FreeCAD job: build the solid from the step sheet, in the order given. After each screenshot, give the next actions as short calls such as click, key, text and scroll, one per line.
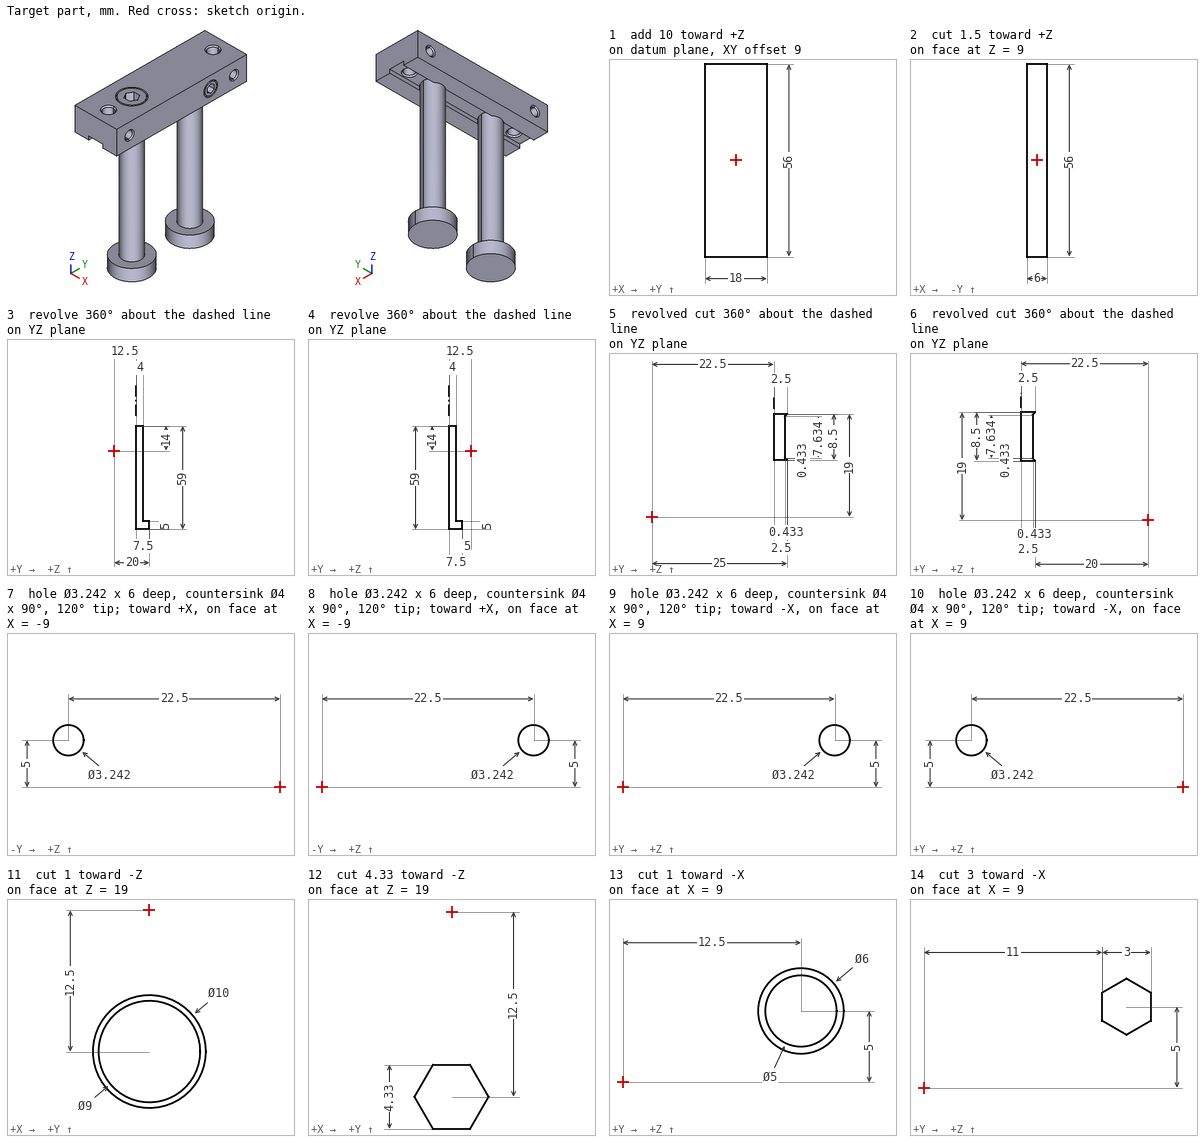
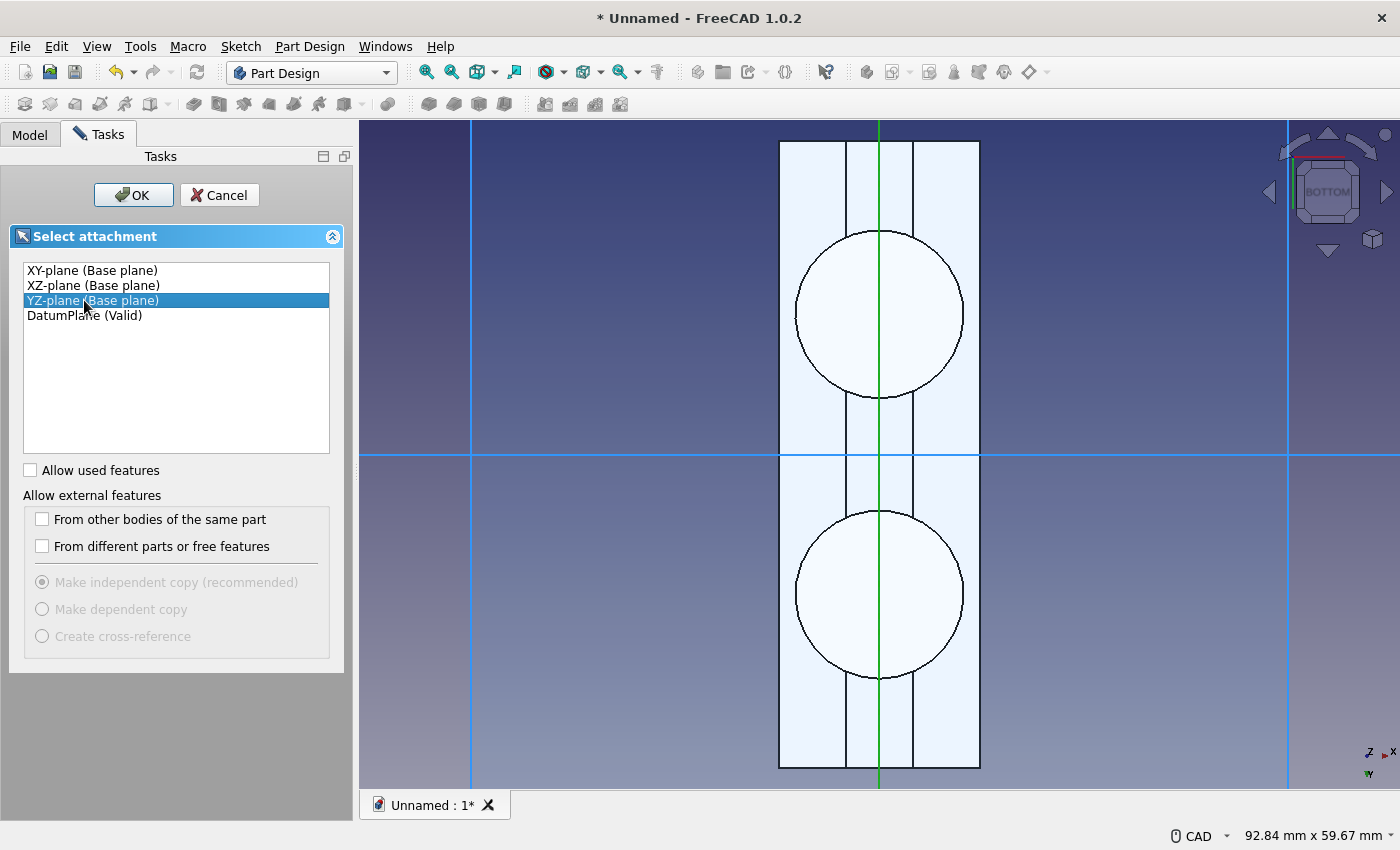
click(134, 195)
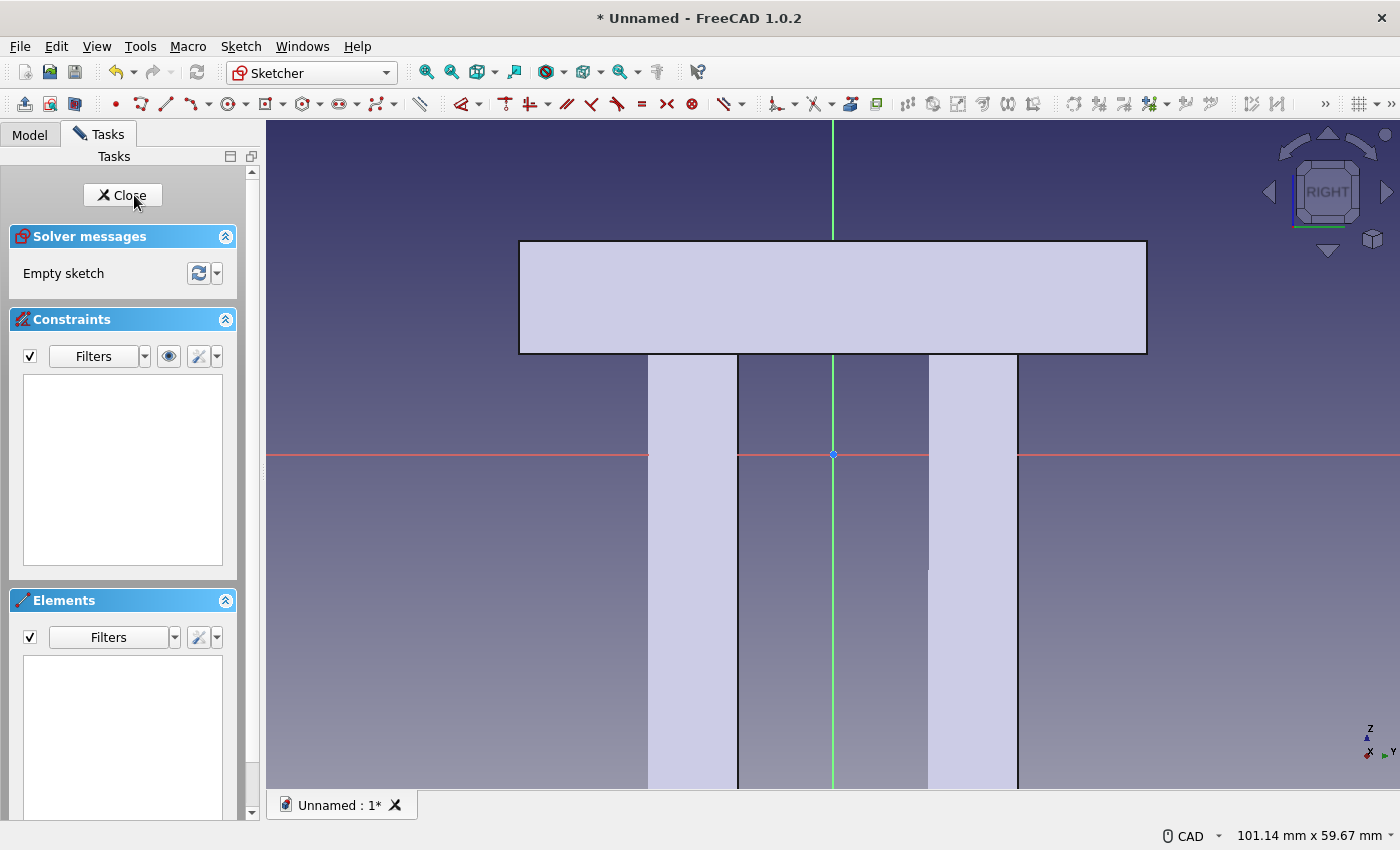
click(75, 104)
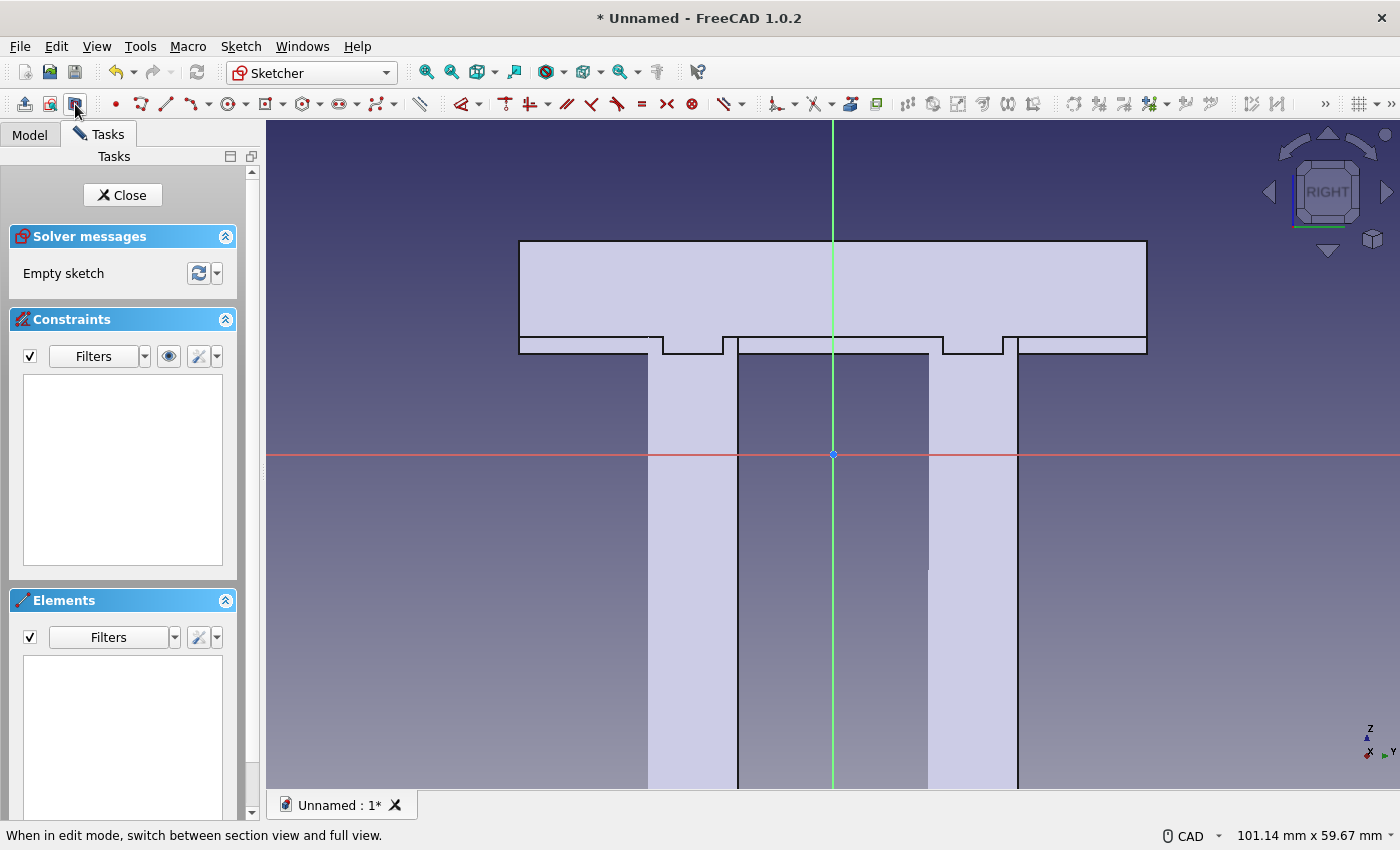
scroll(1227, 176, up, 3)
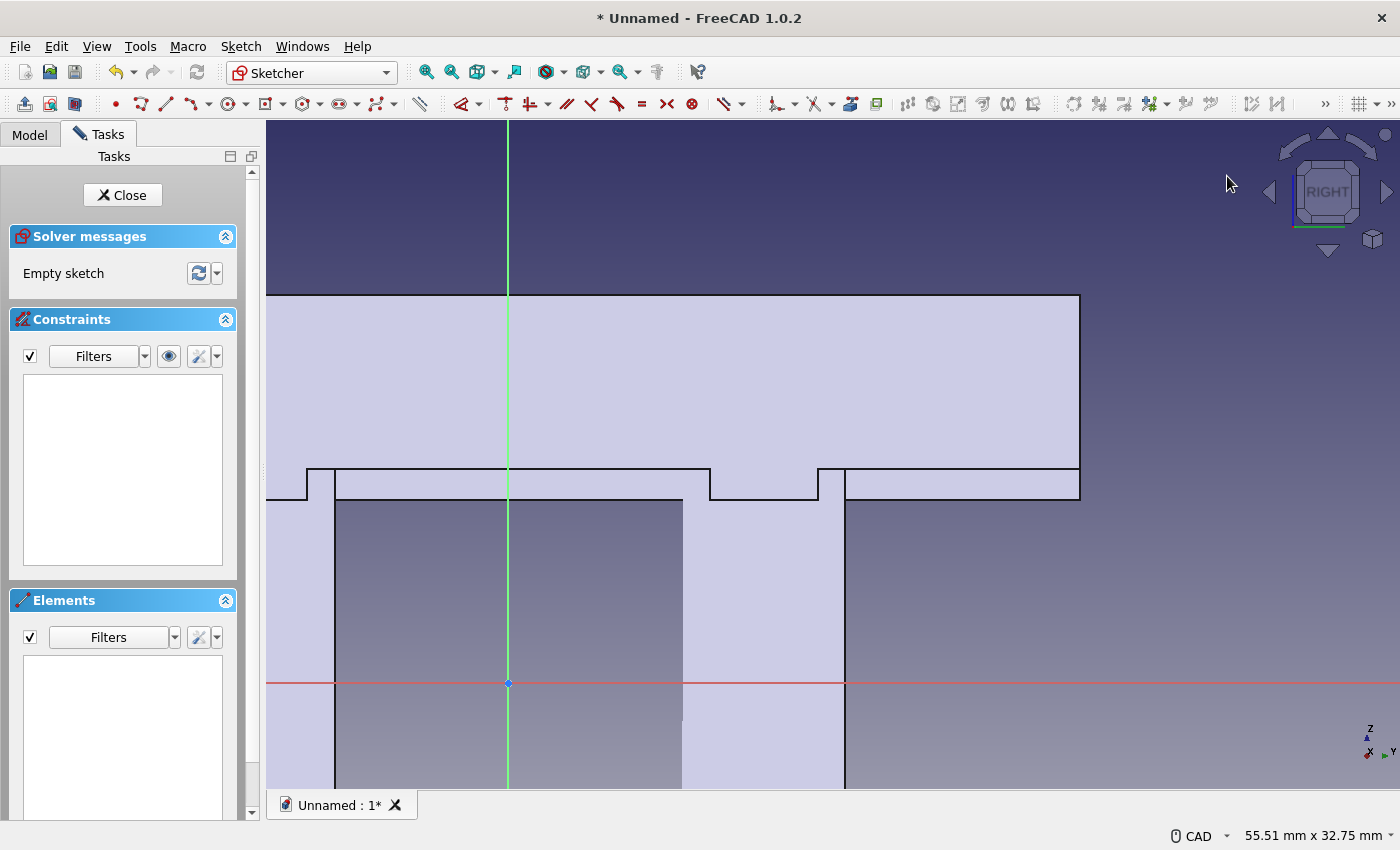
click(141, 104)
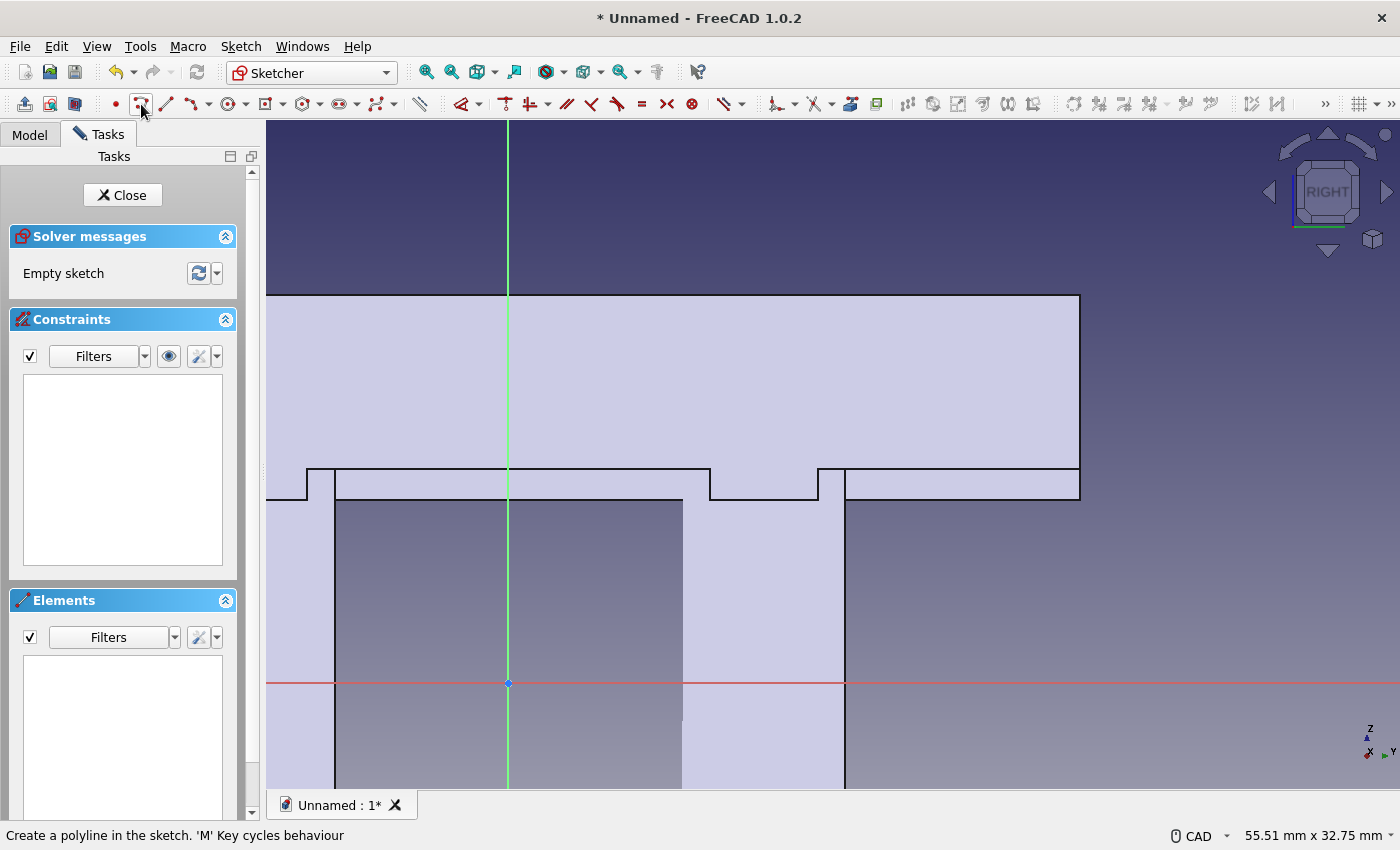
click(968, 469)
click(1019, 469)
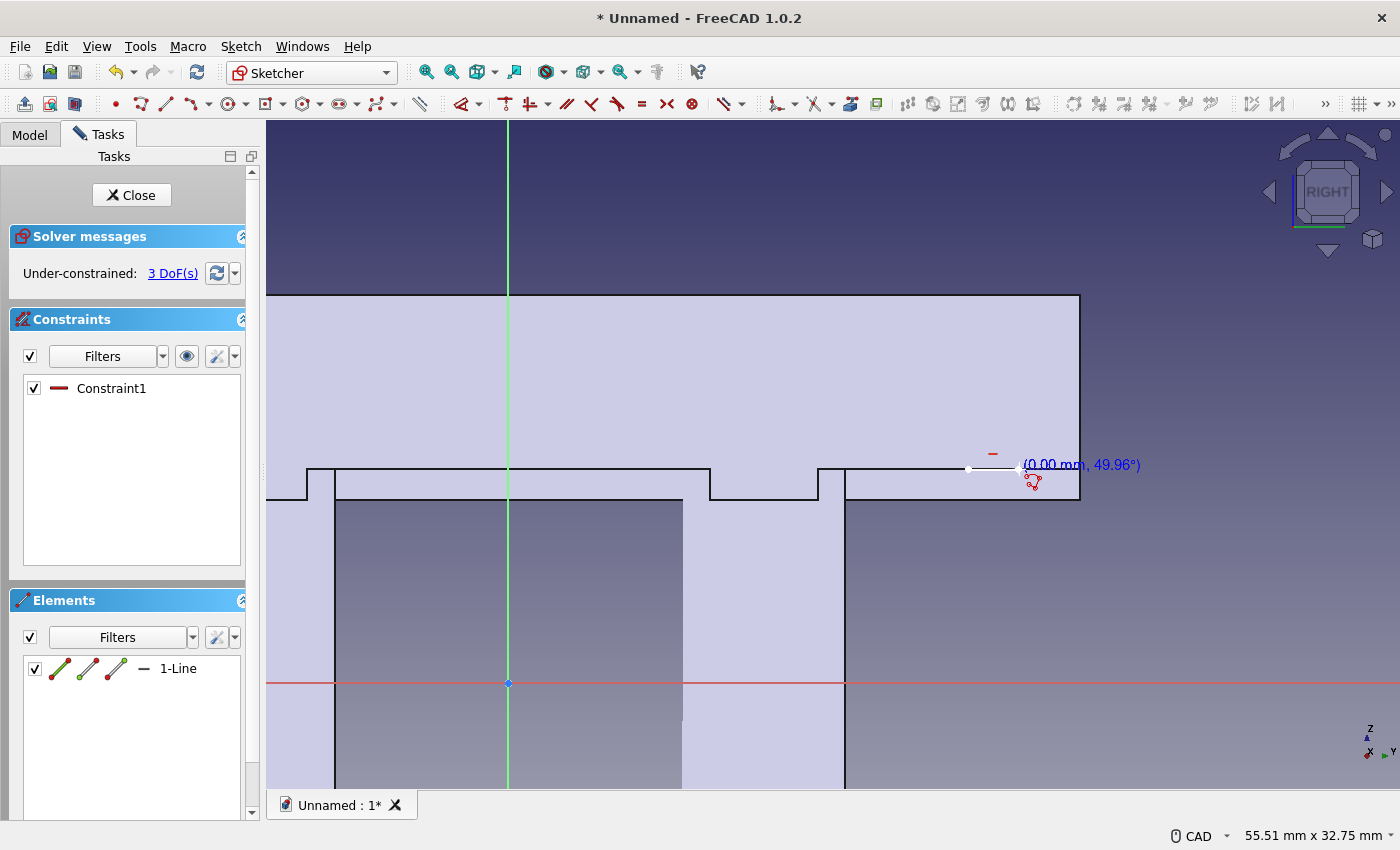
scroll(1010, 460, up, 3)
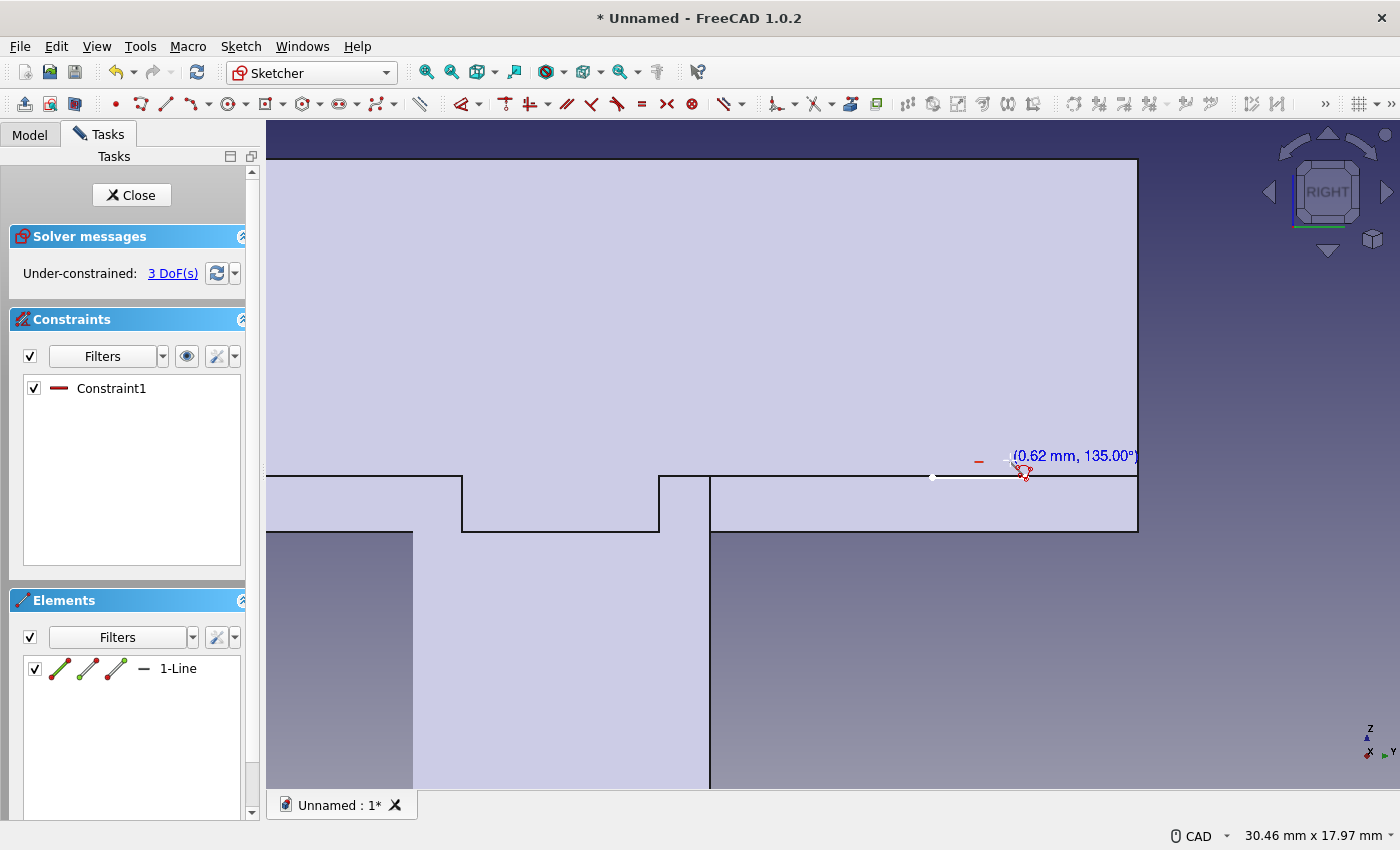
click(1010, 460)
click(1010, 175)
click(1026, 159)
click(933, 159)
click(933, 478)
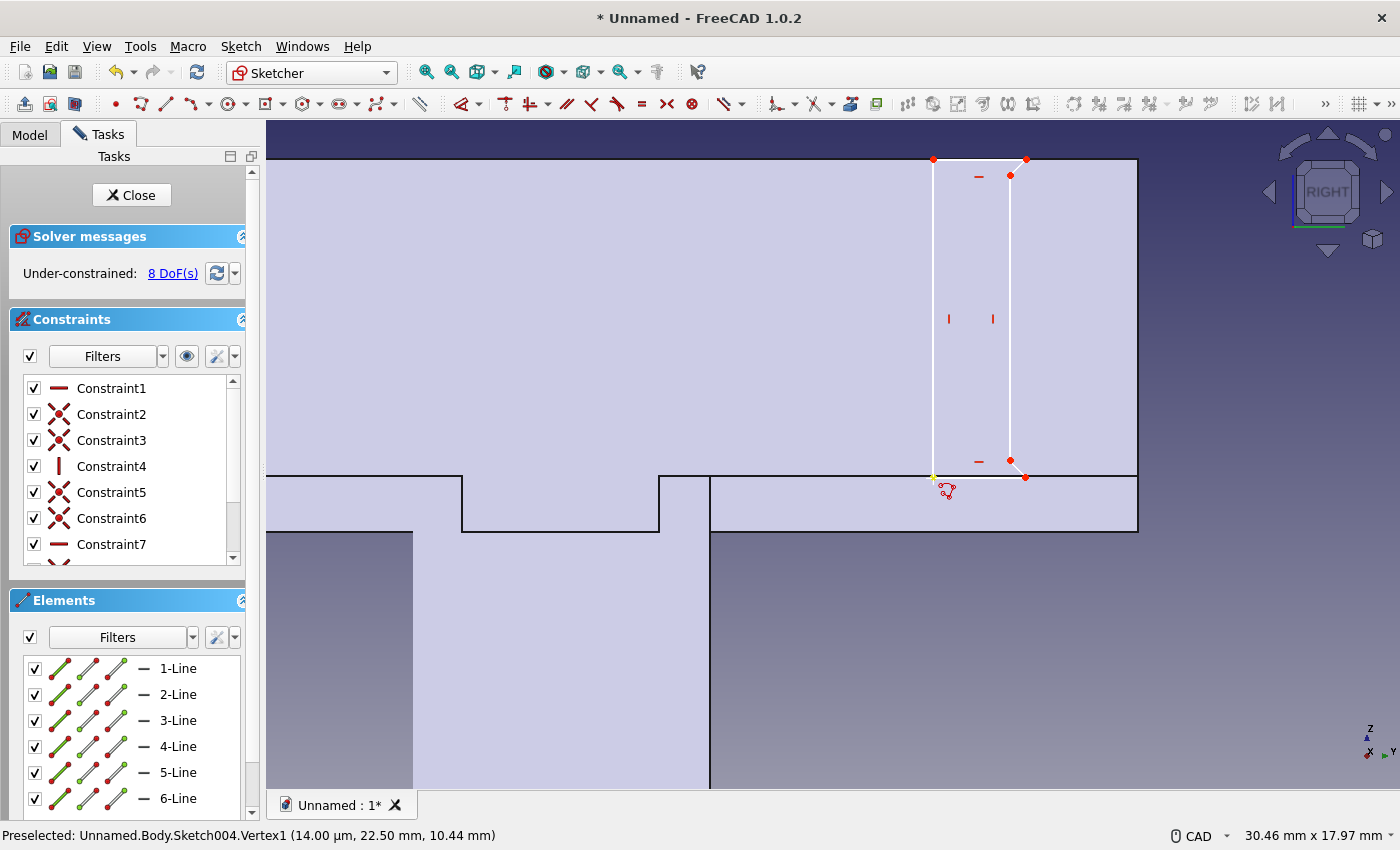
click(166, 104)